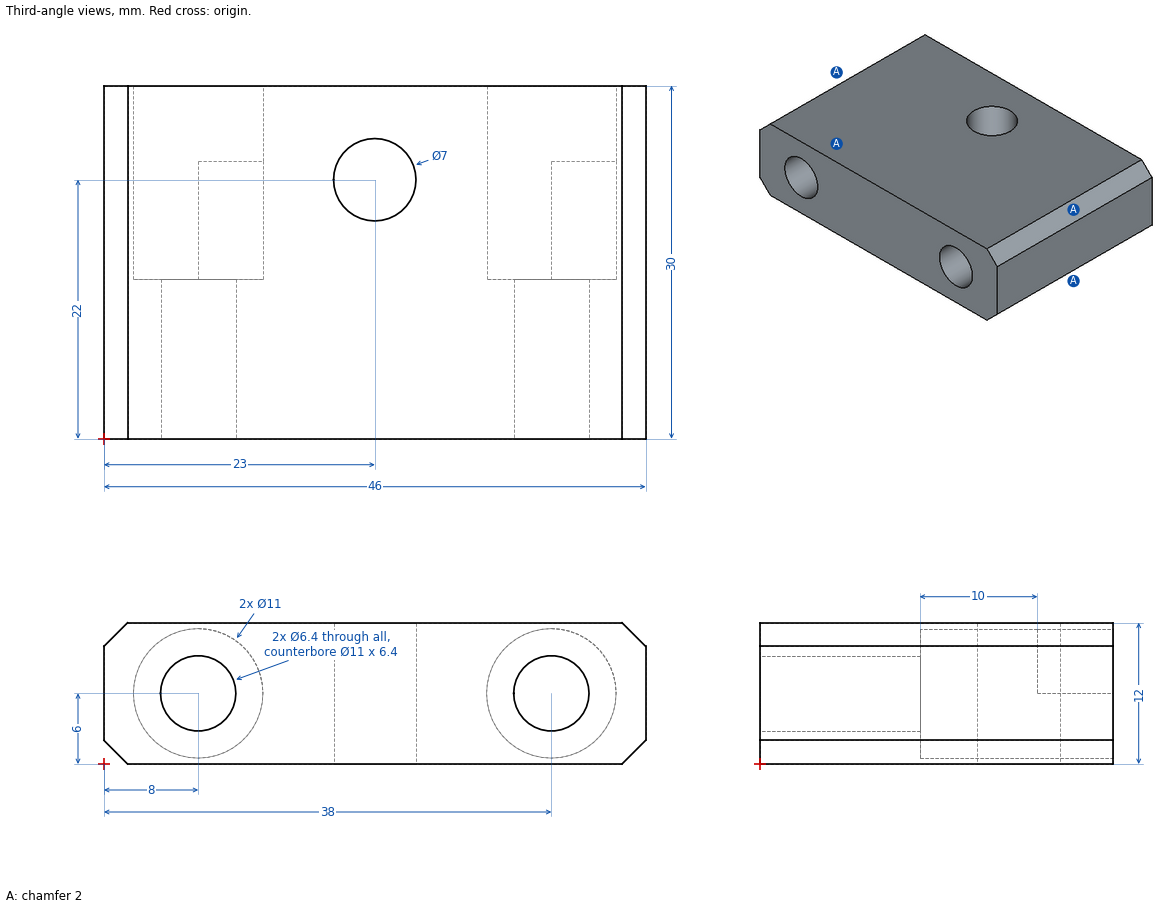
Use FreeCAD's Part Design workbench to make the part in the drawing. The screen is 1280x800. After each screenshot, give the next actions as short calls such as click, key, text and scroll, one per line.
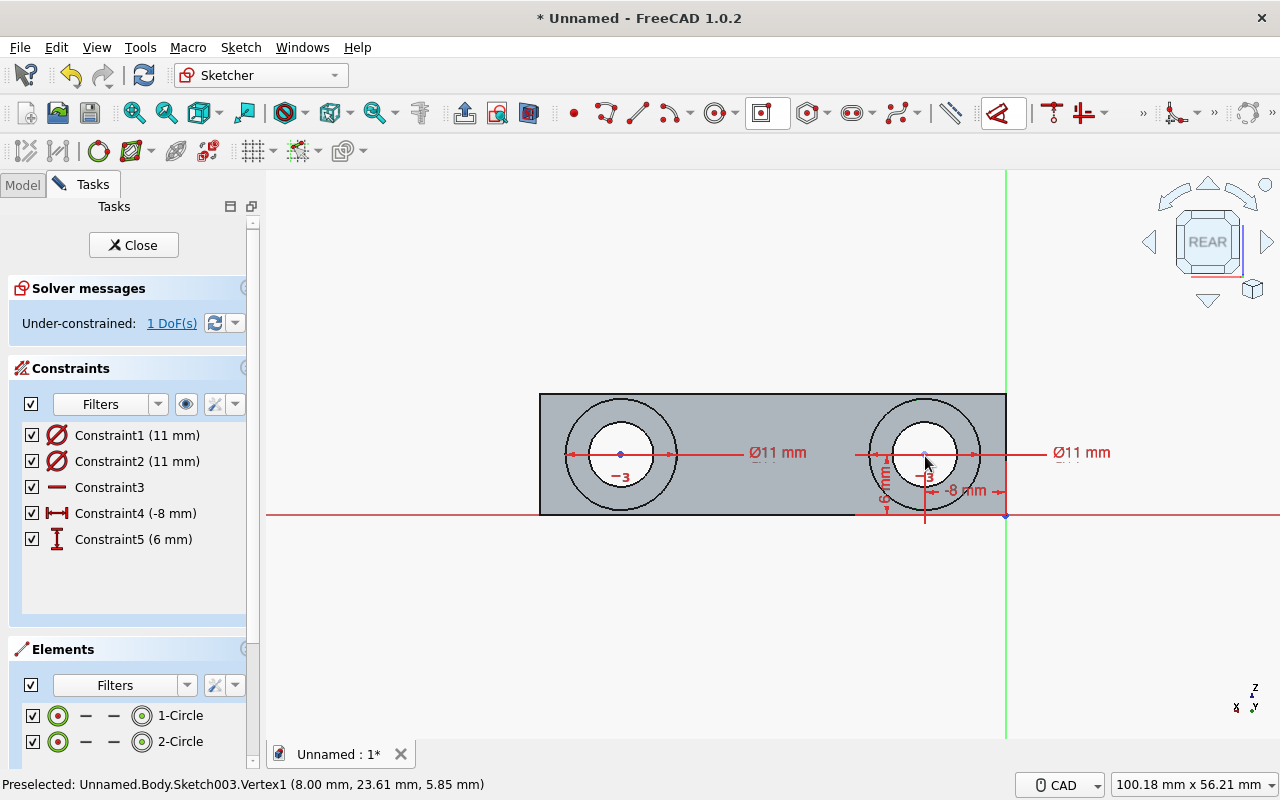
click(621, 455)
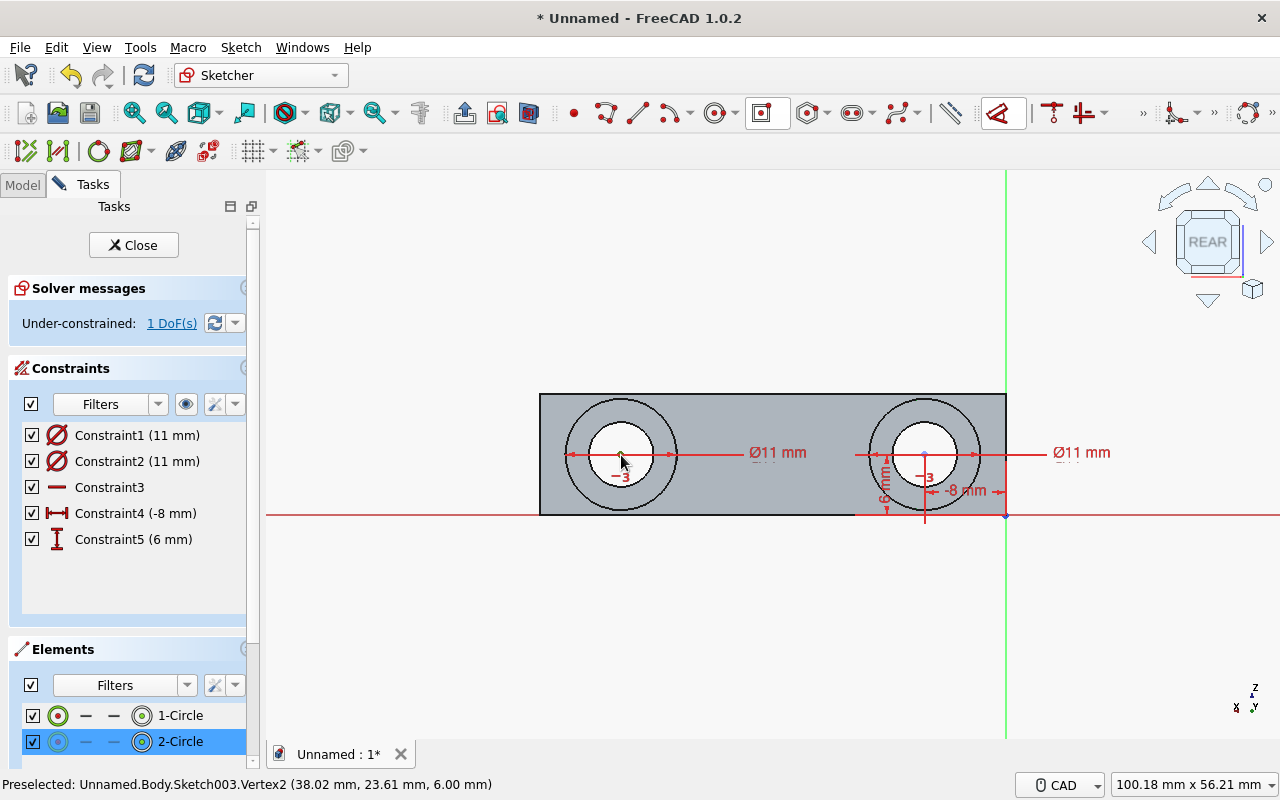
key(l)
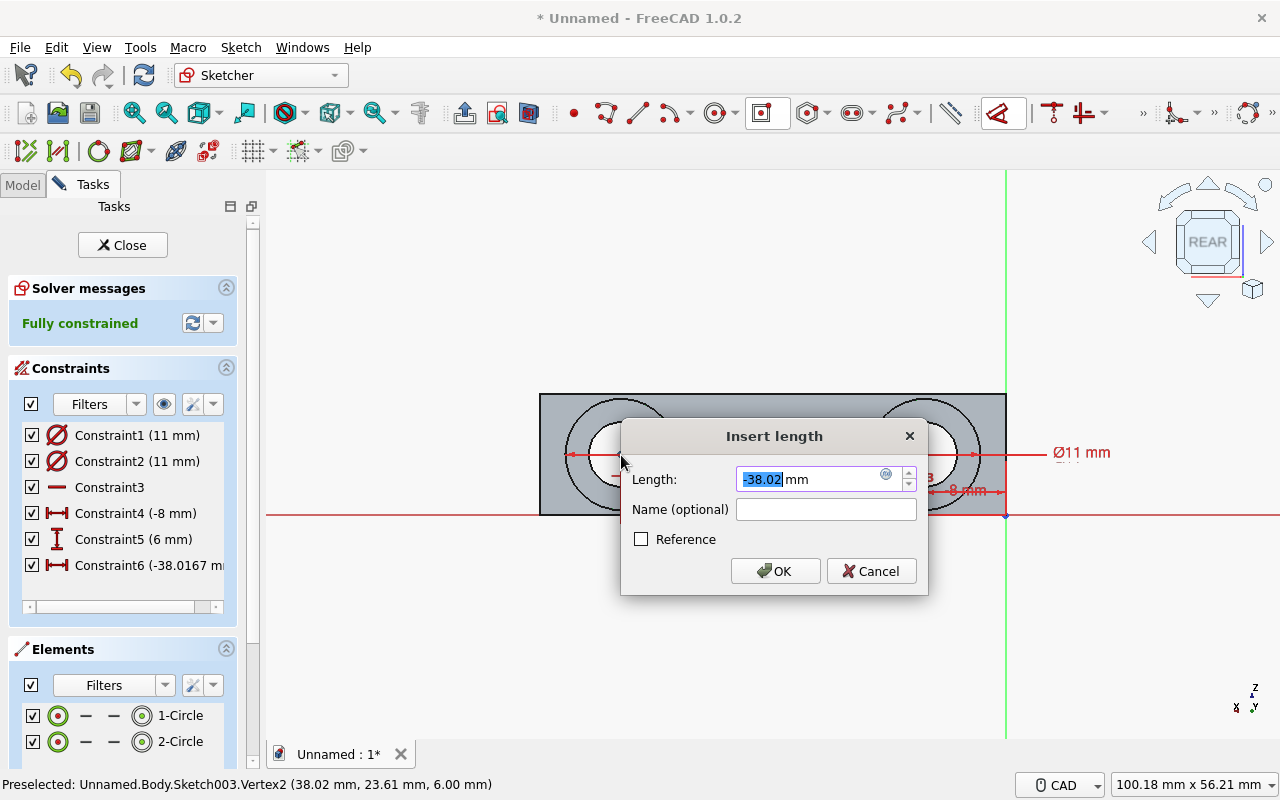
text(-38)
key(Return)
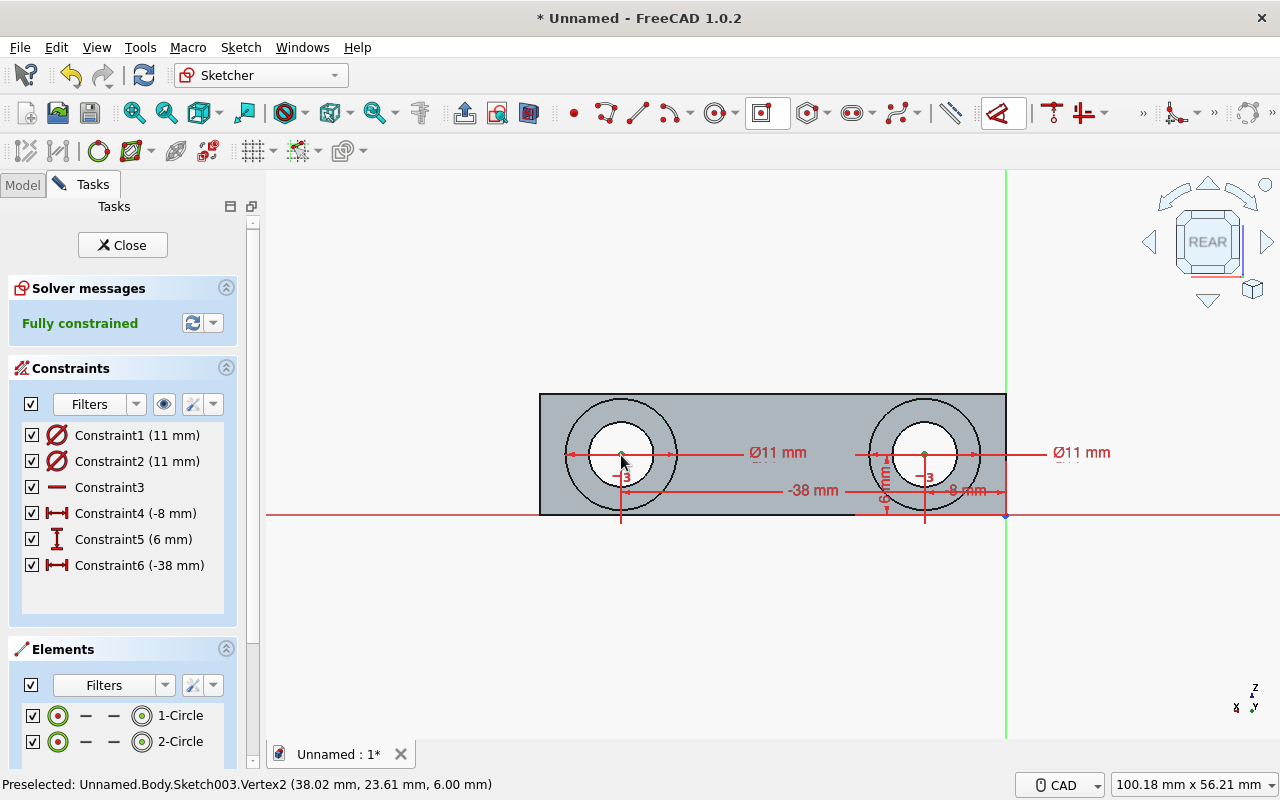
click(123, 245)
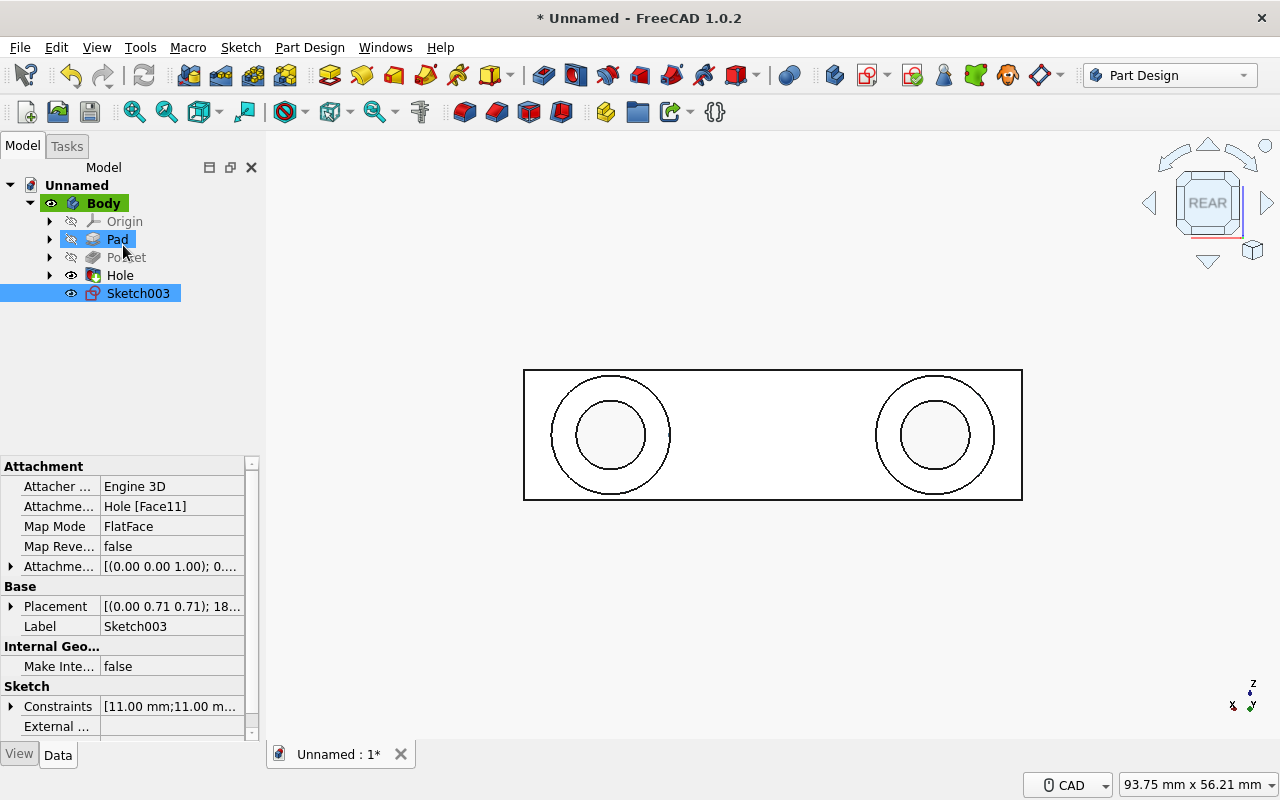
click(544, 76)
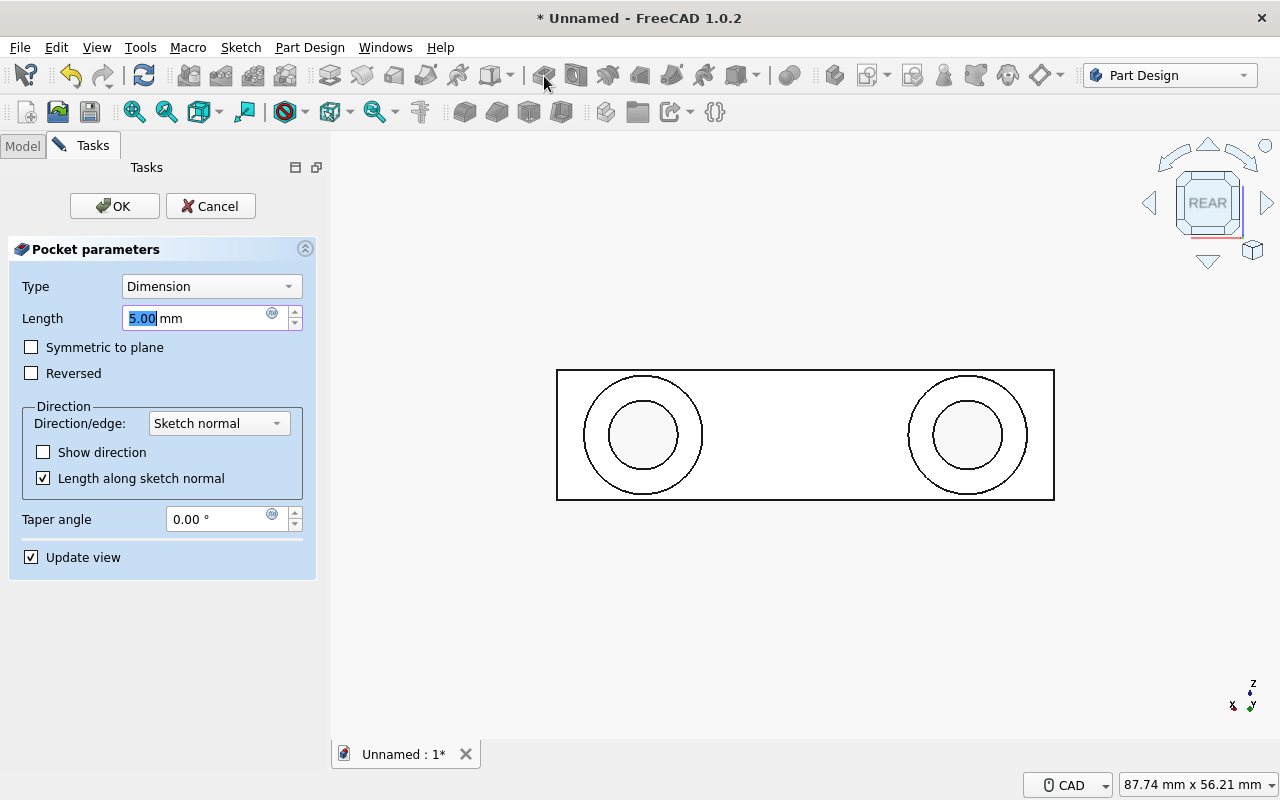
text(10)
key(Tab)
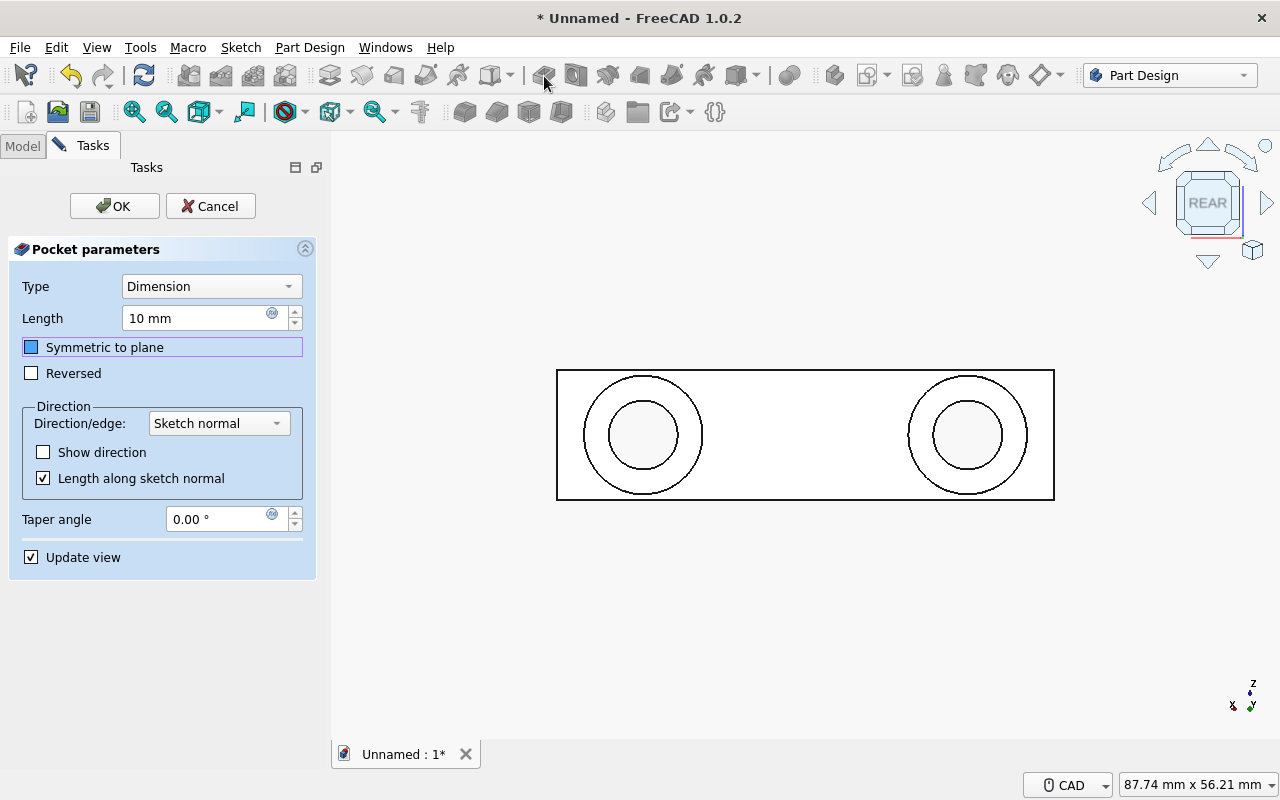
click(115, 206)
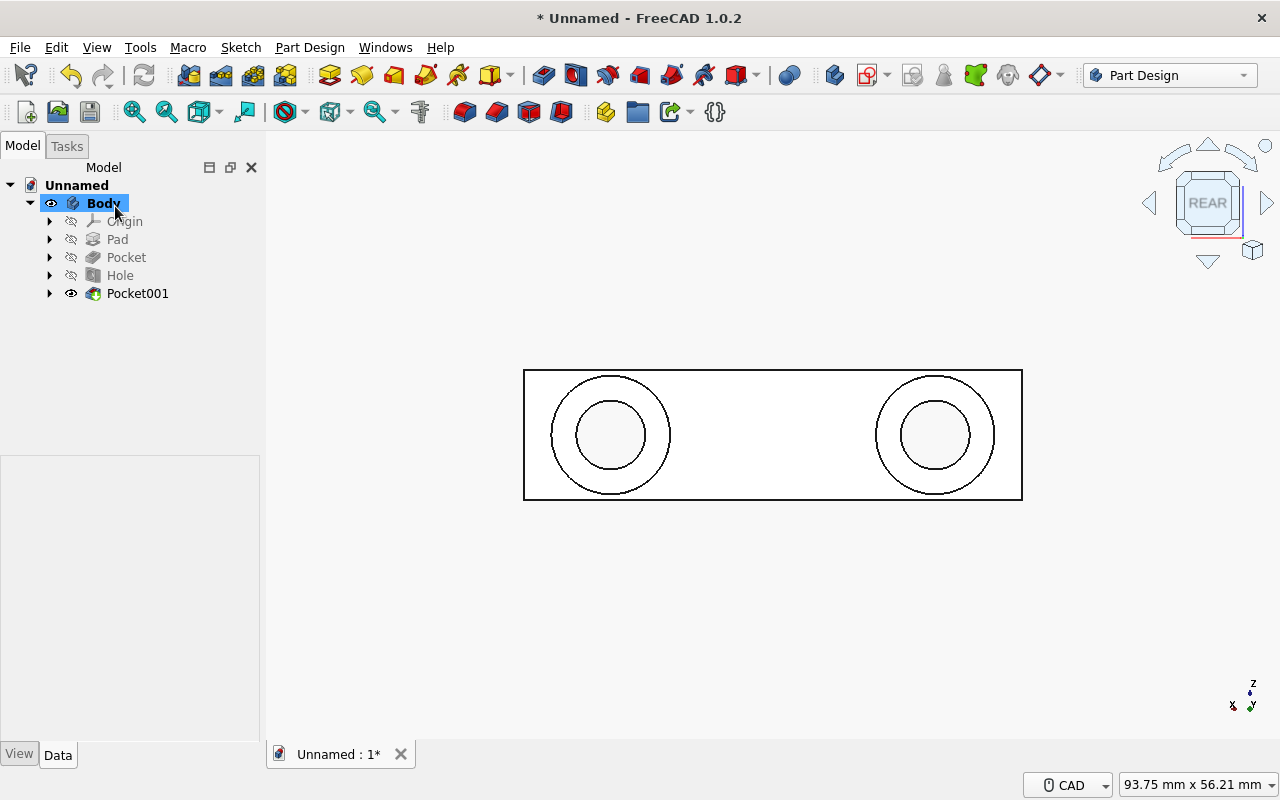
key(0)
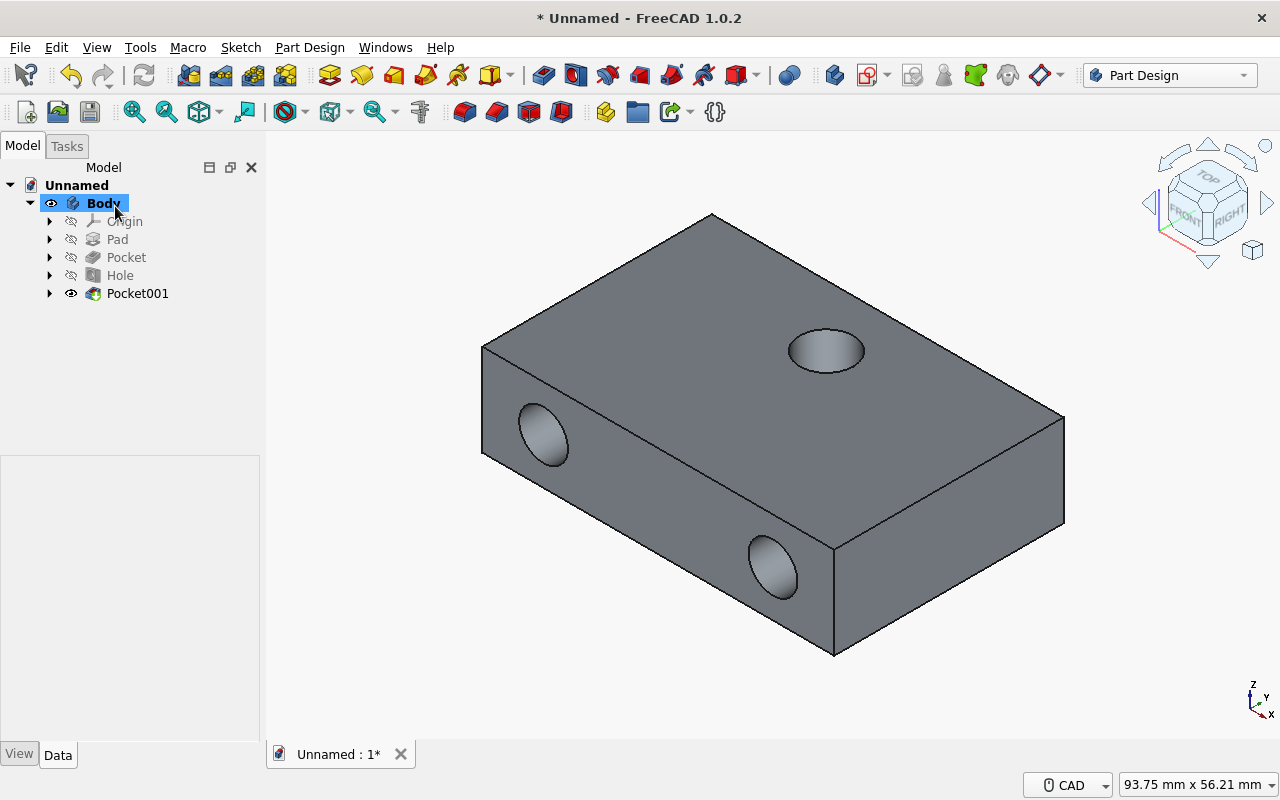
click(949, 483)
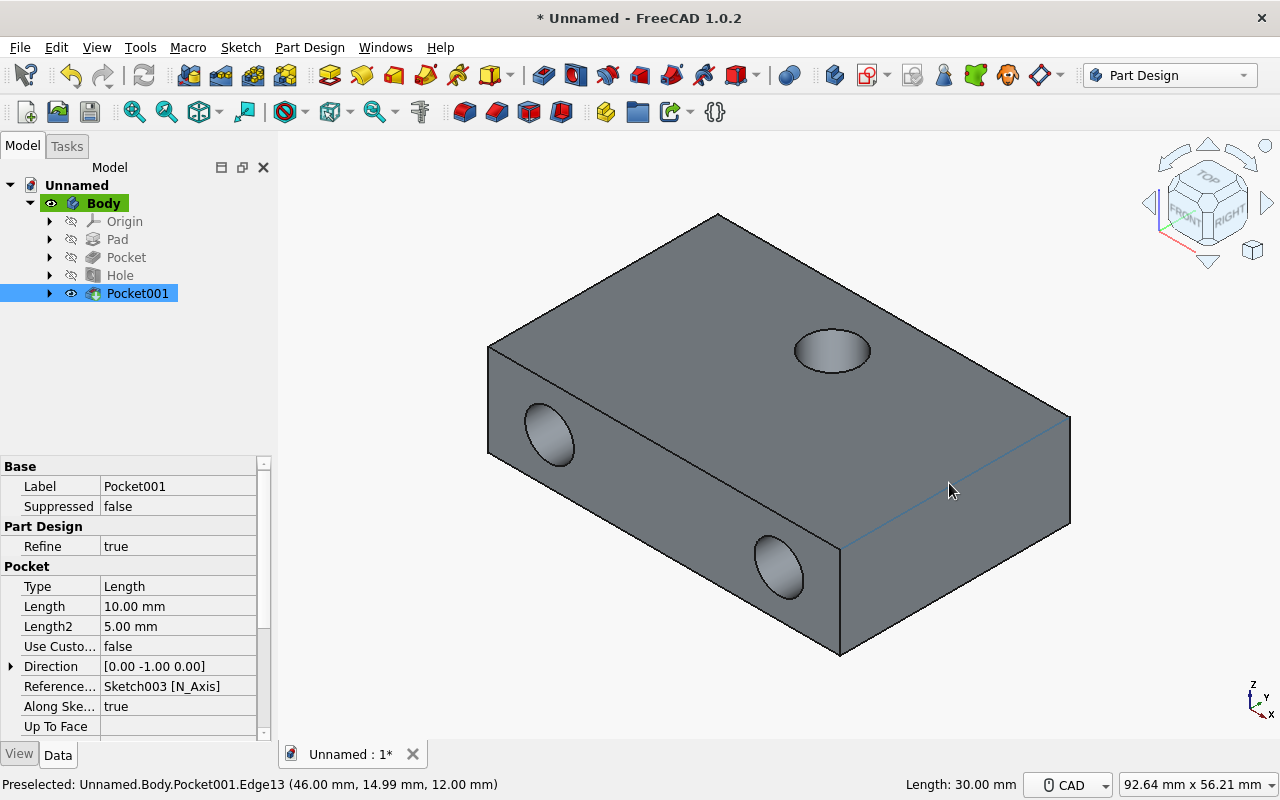
key(2)